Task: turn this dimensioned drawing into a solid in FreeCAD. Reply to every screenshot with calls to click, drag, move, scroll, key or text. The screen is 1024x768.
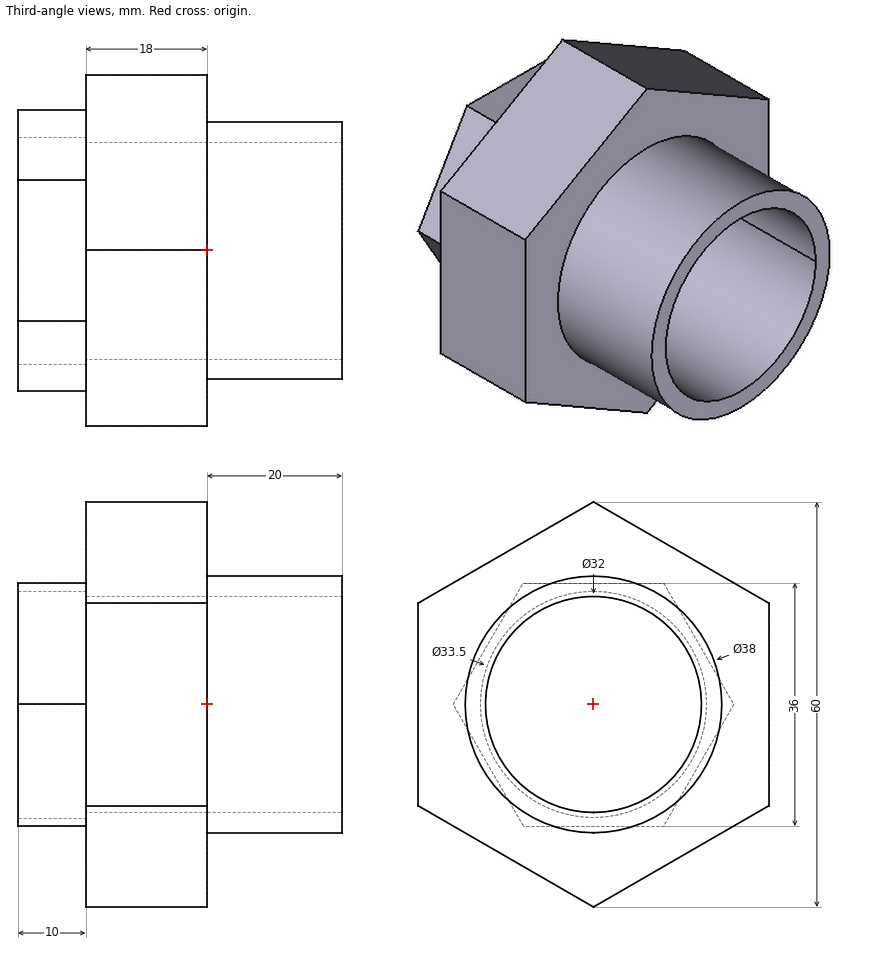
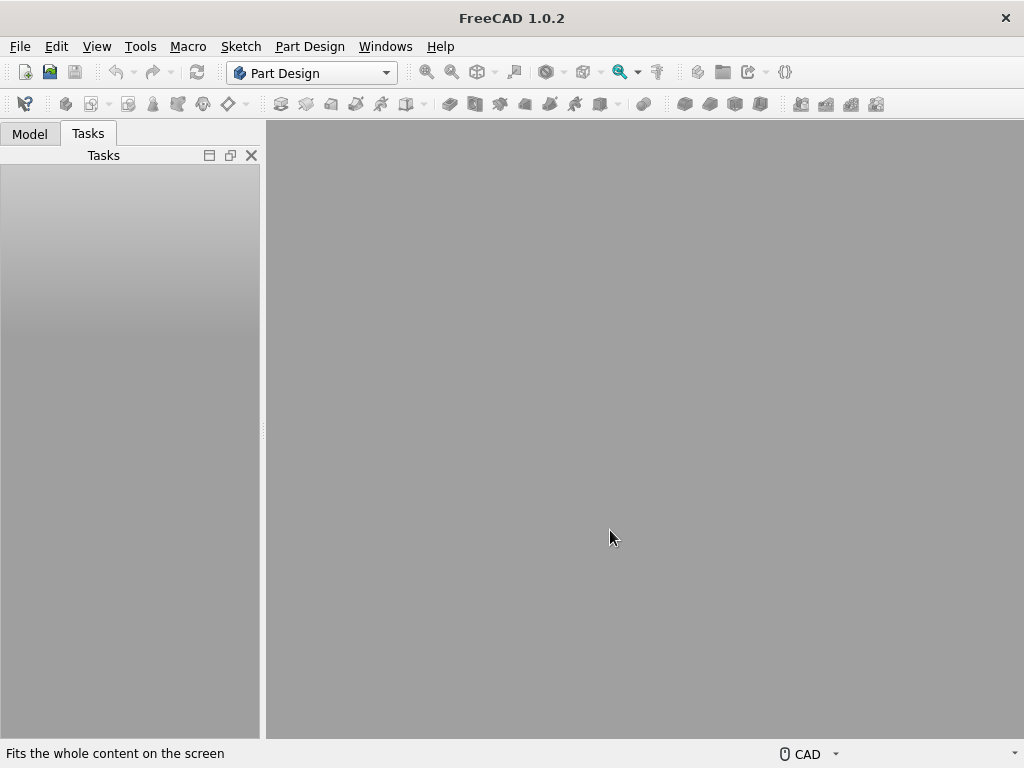
click(25, 72)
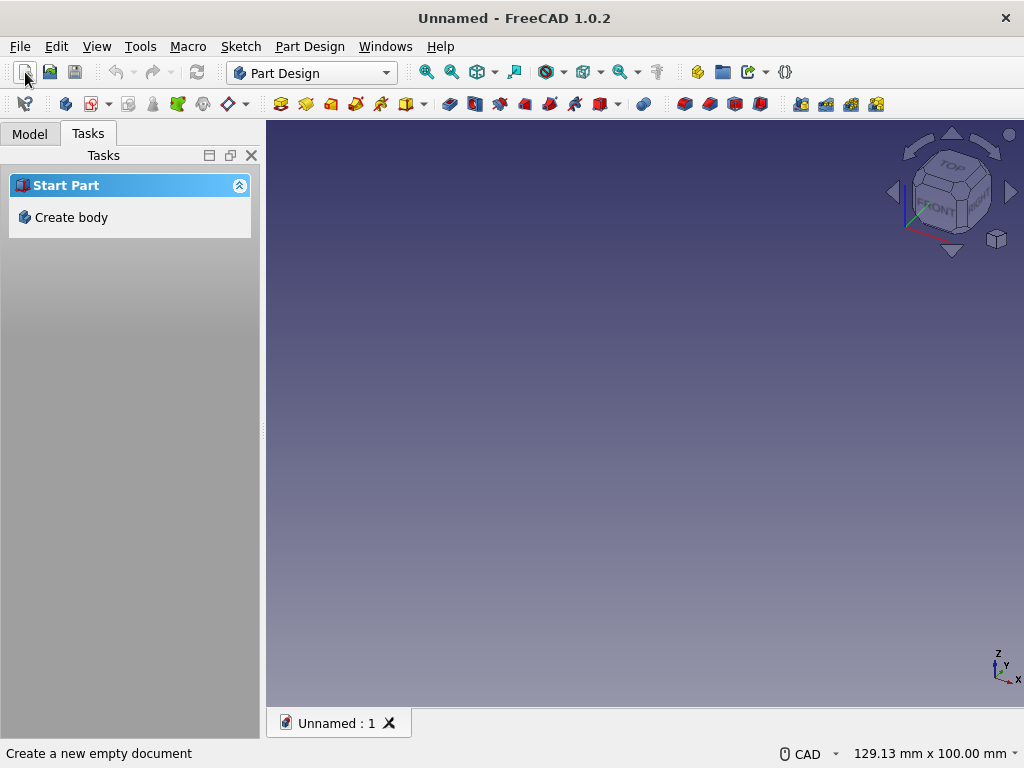
click(90, 104)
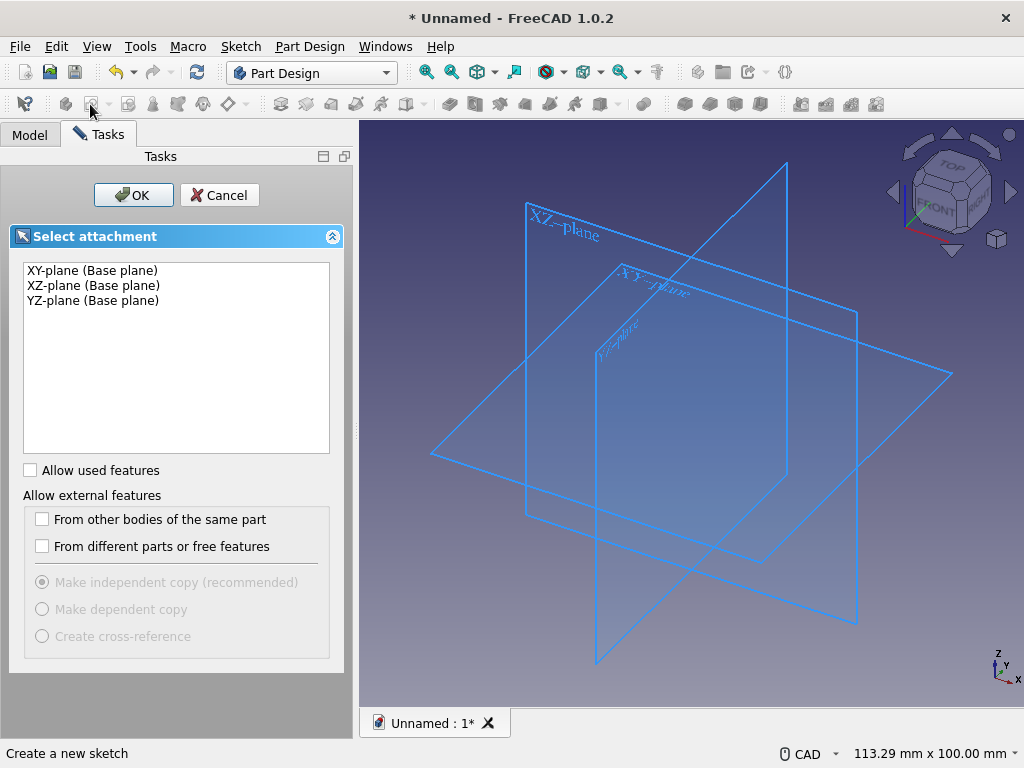
click(84, 300)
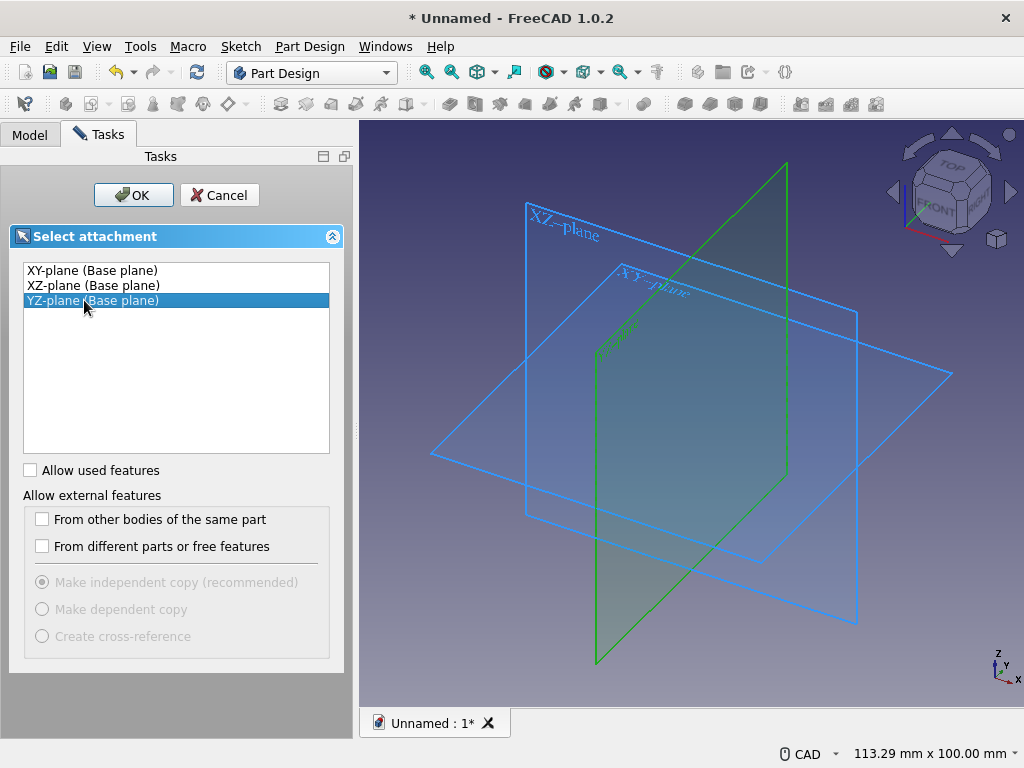
click(134, 195)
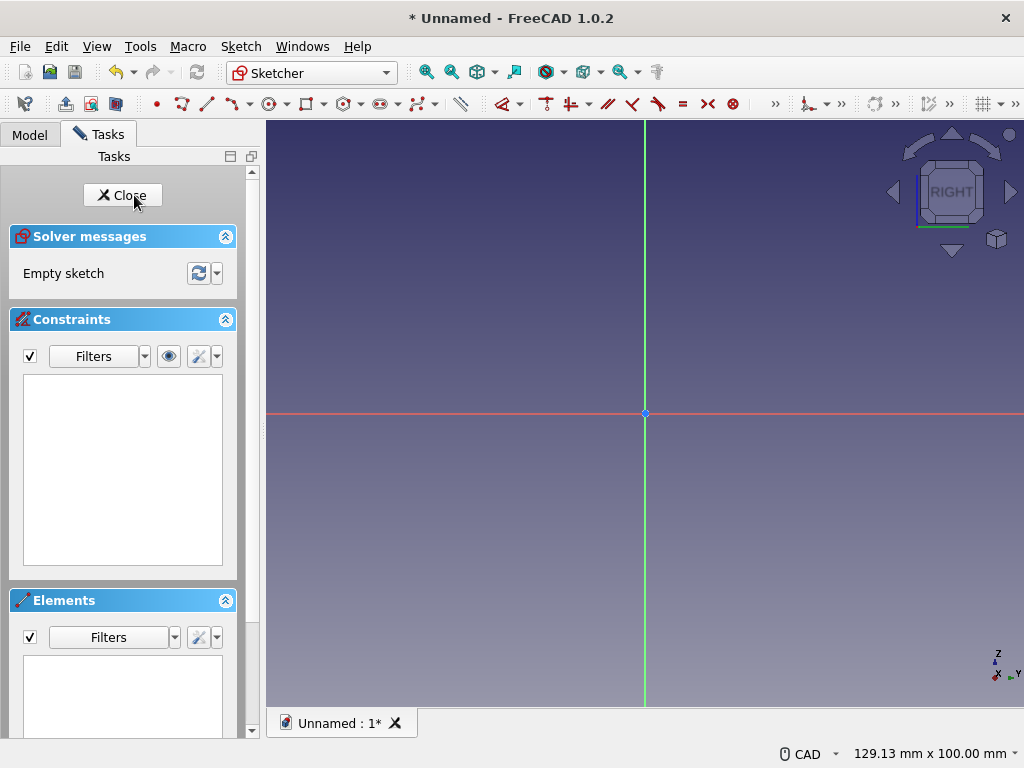
scroll(728, 414, up, 3)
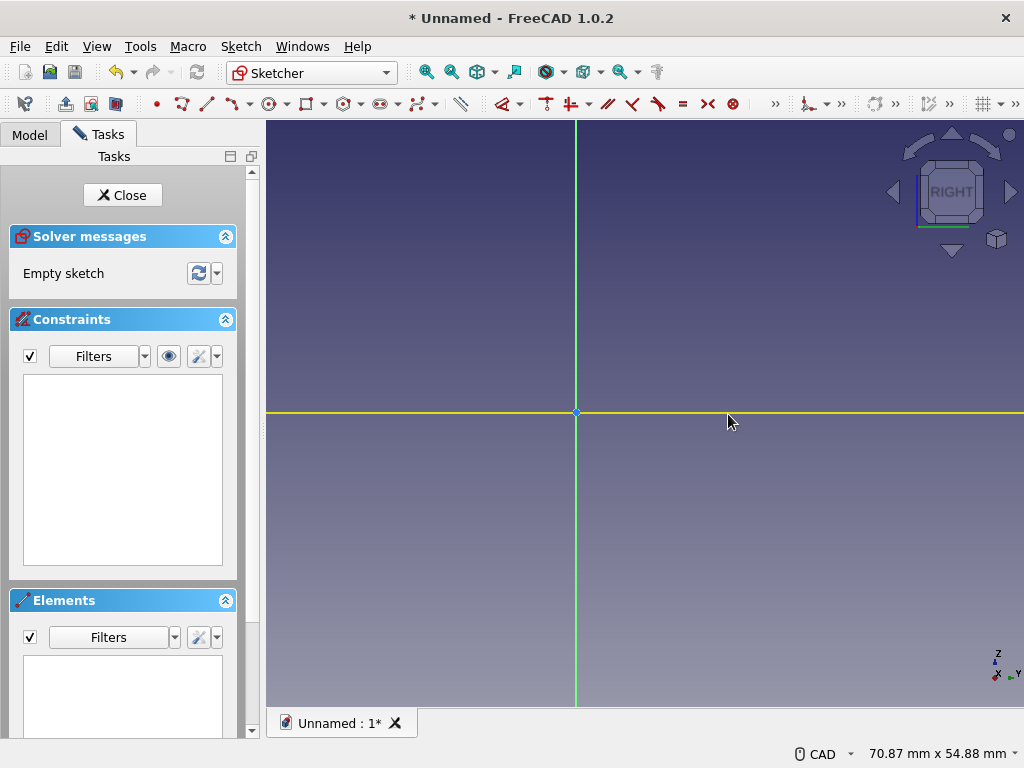
key(g)
key(c)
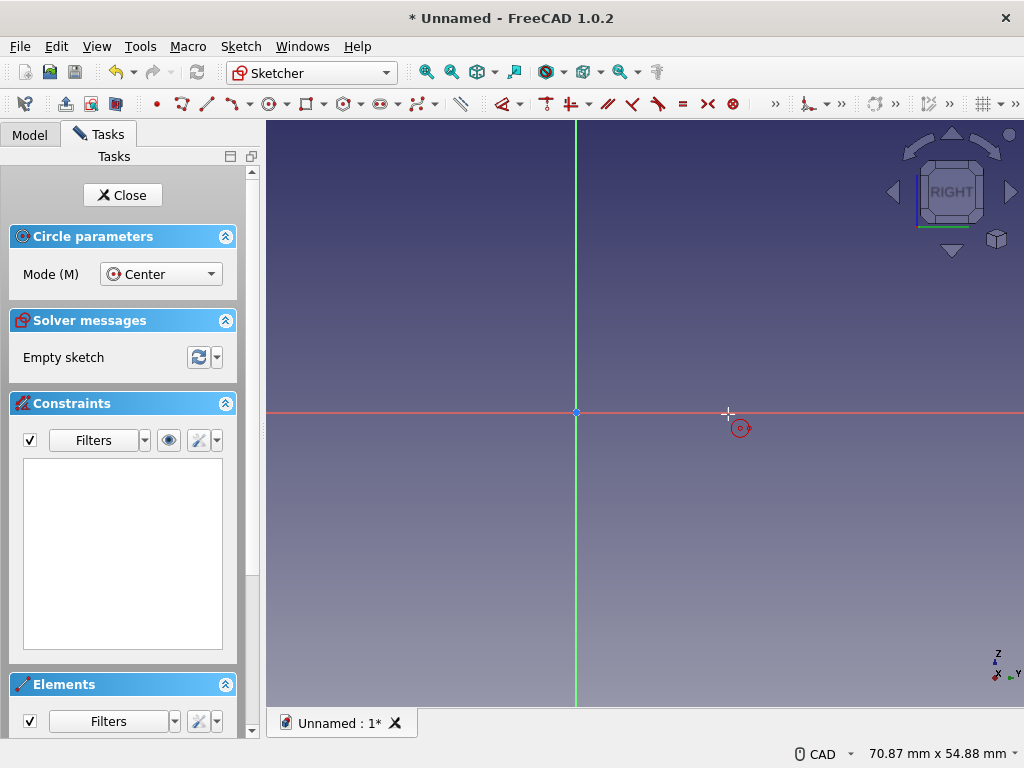
click(576, 413)
click(720, 269)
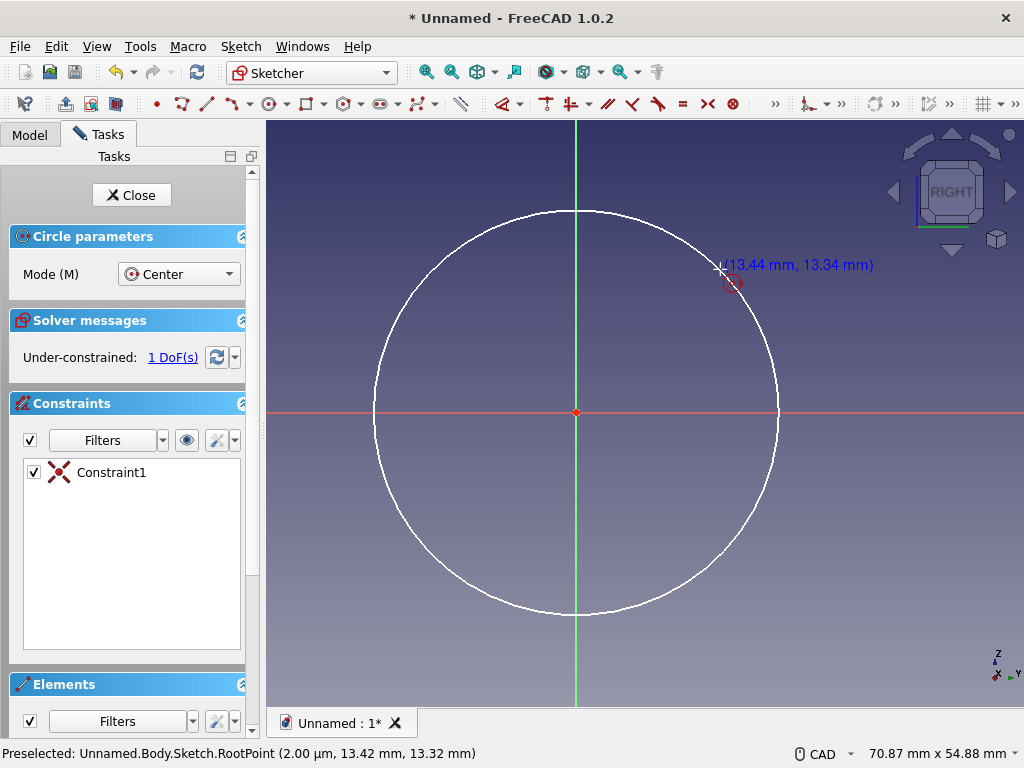
click(576, 413)
click(697, 292)
key(Escape)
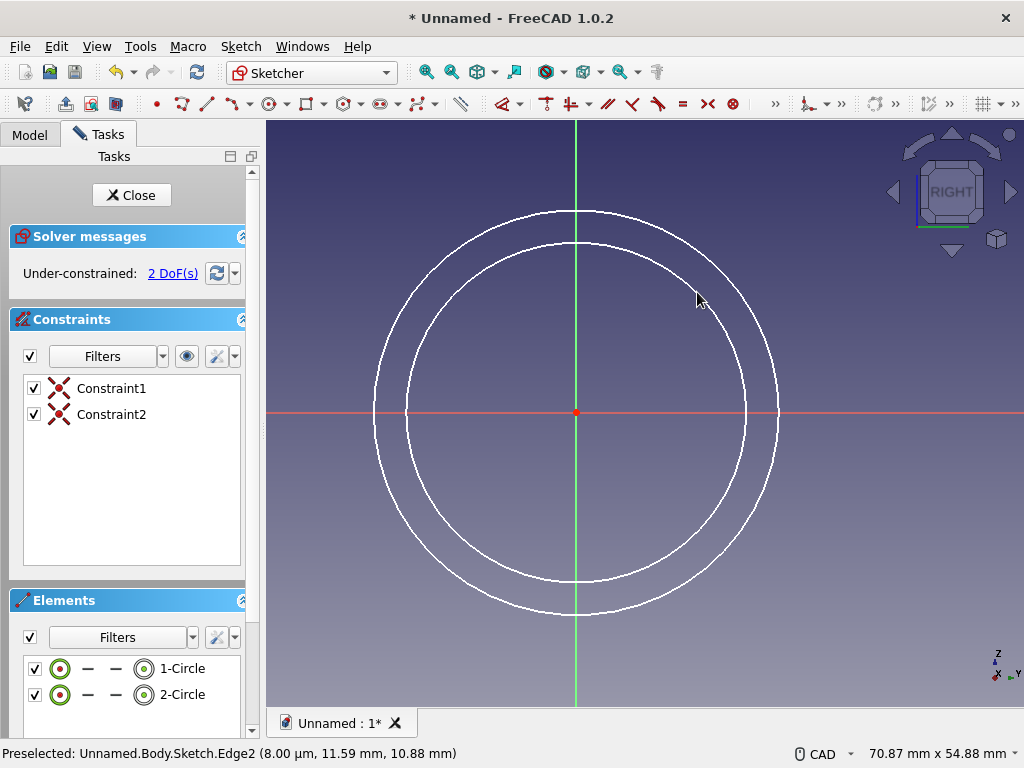
click(719, 269)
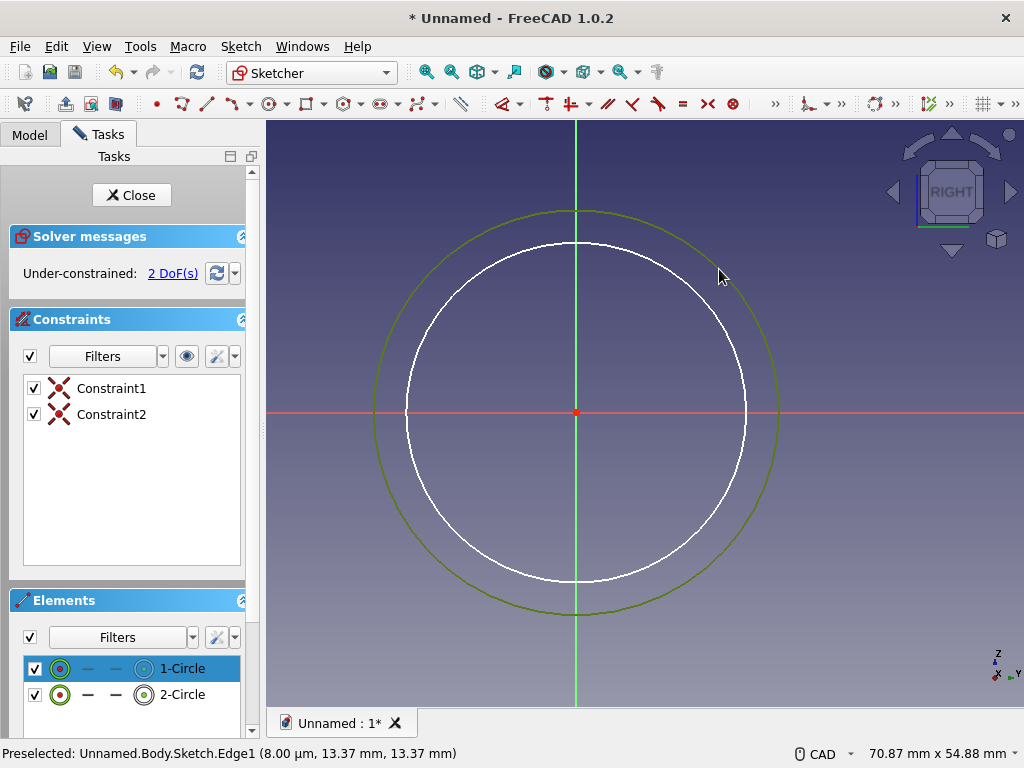
key(k)
key(o)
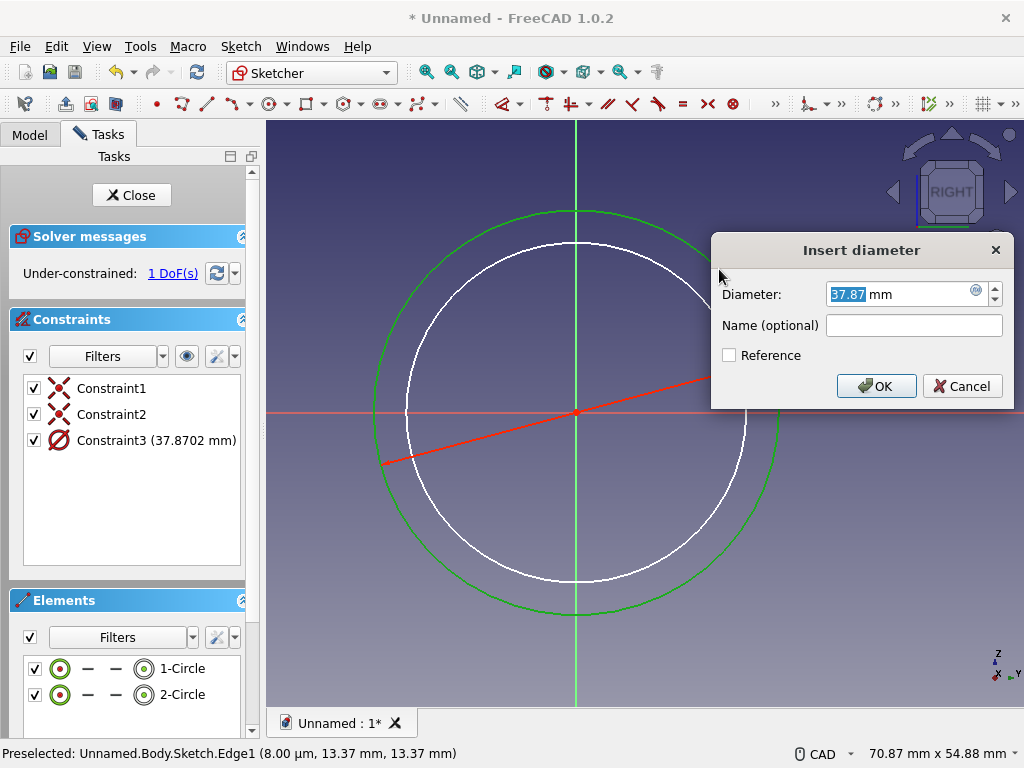
text(38)
key(Return)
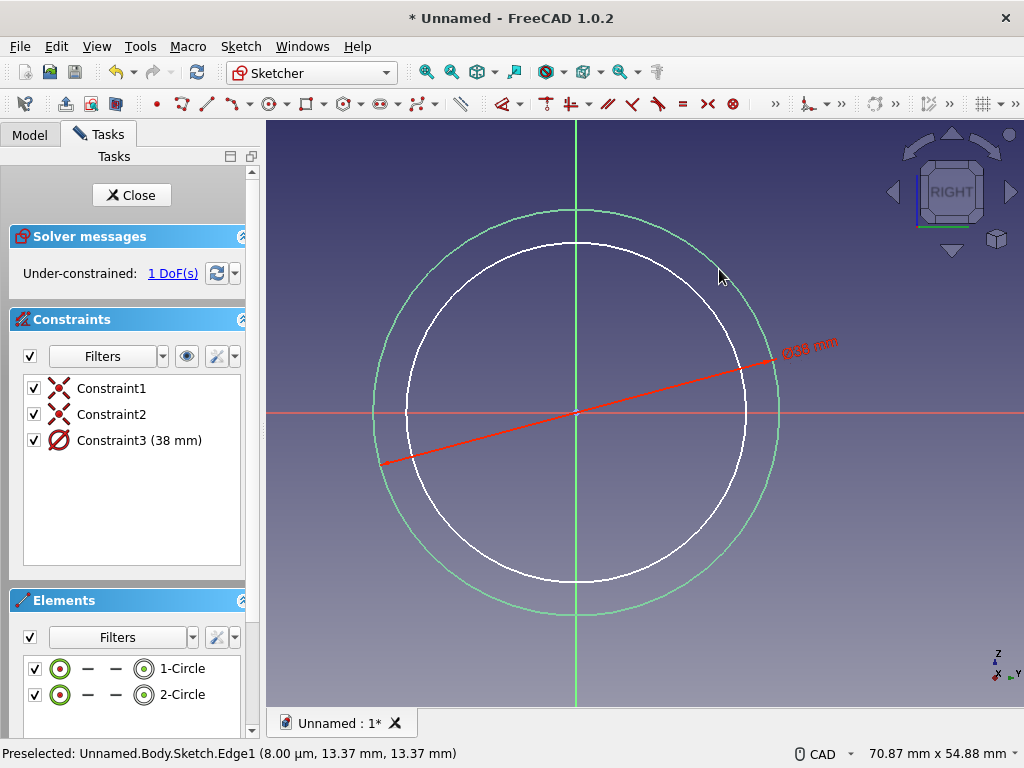
click(696, 292)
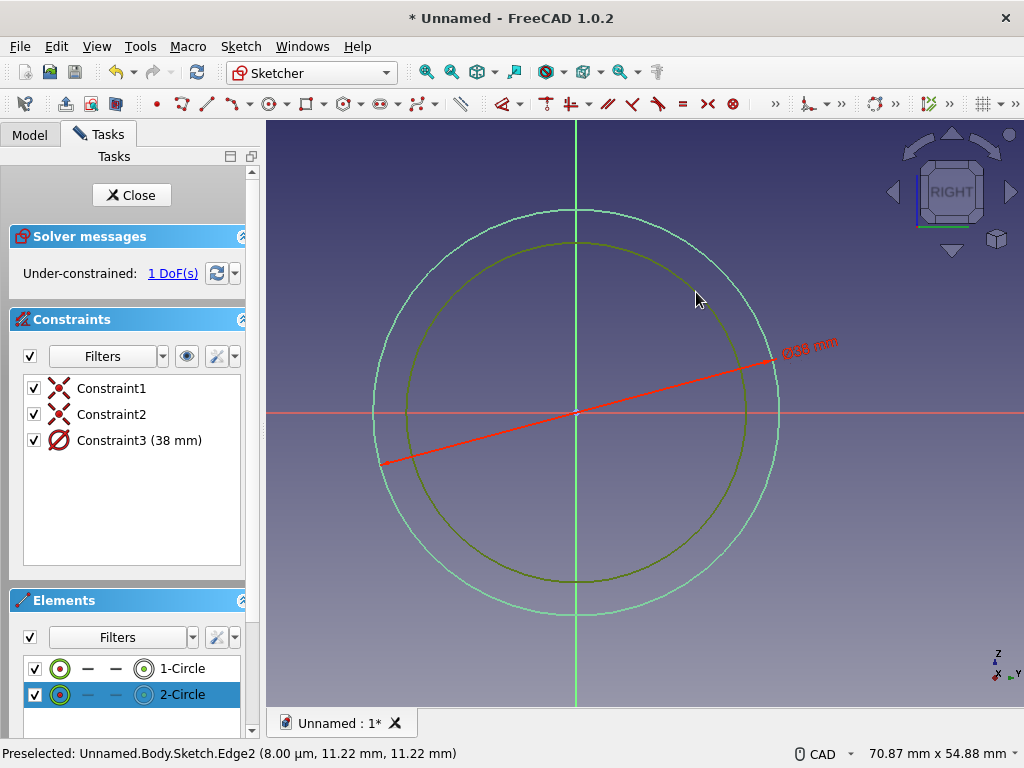
key(k)
key(o)